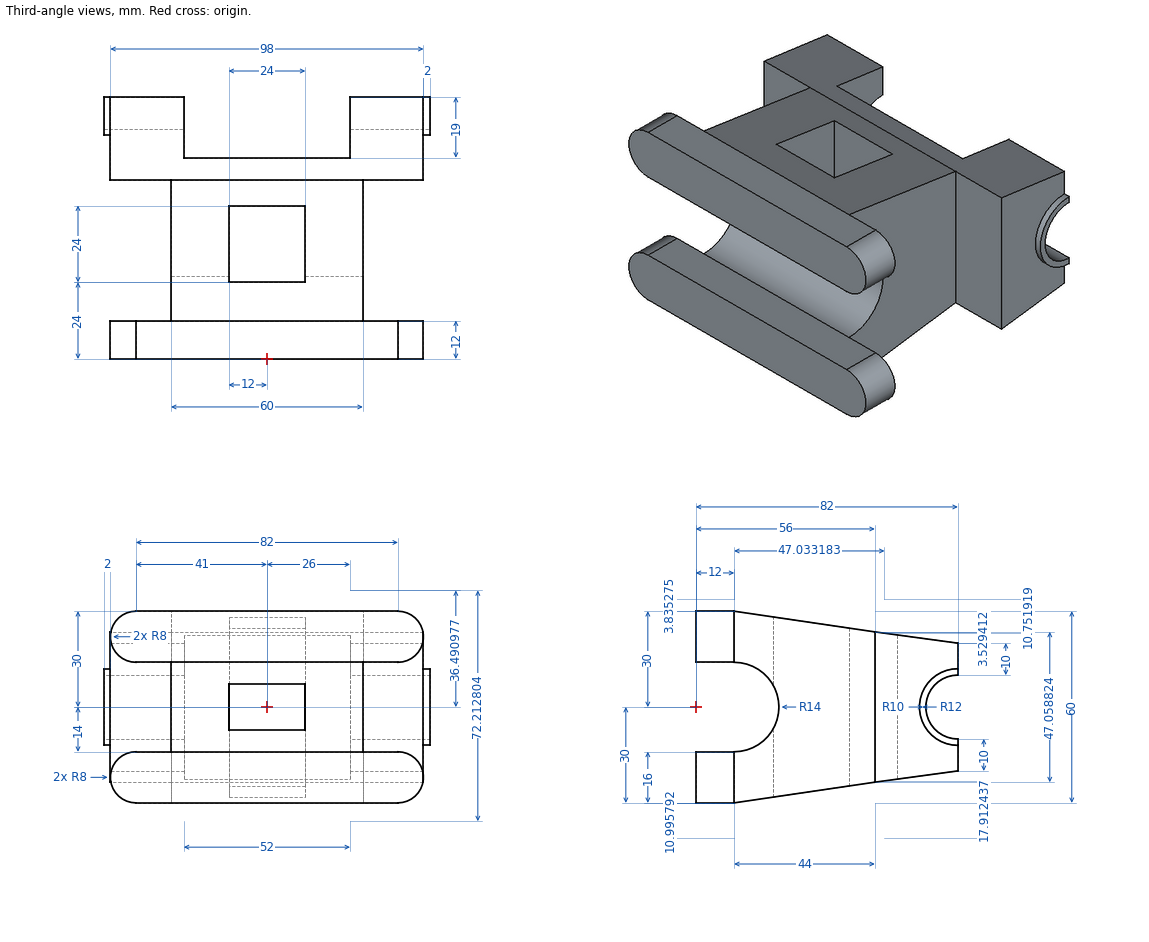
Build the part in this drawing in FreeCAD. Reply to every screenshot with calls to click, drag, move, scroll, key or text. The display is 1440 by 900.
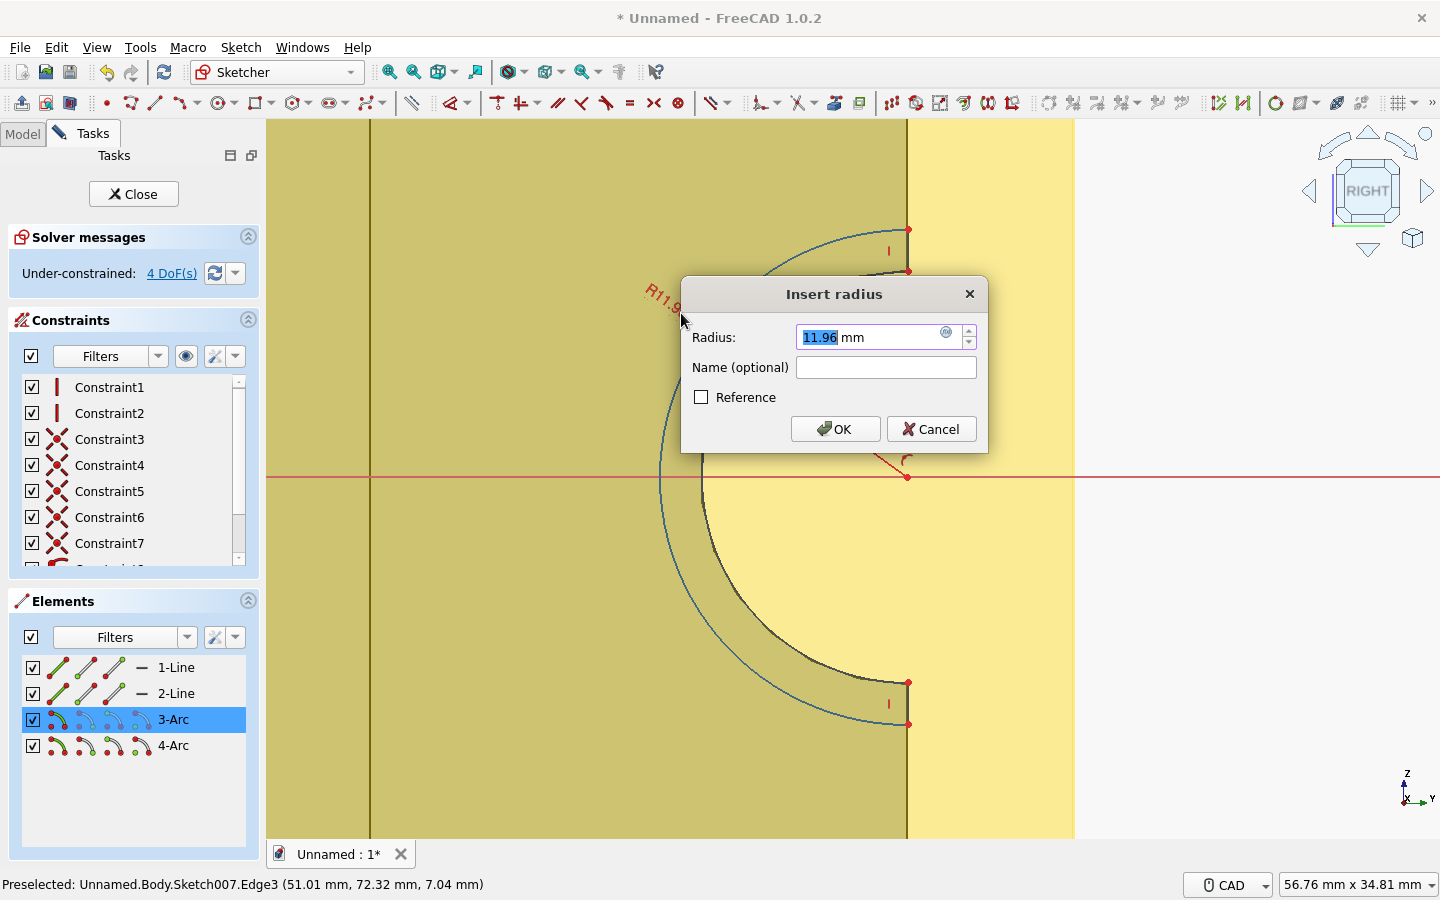
text(12)
key(Return)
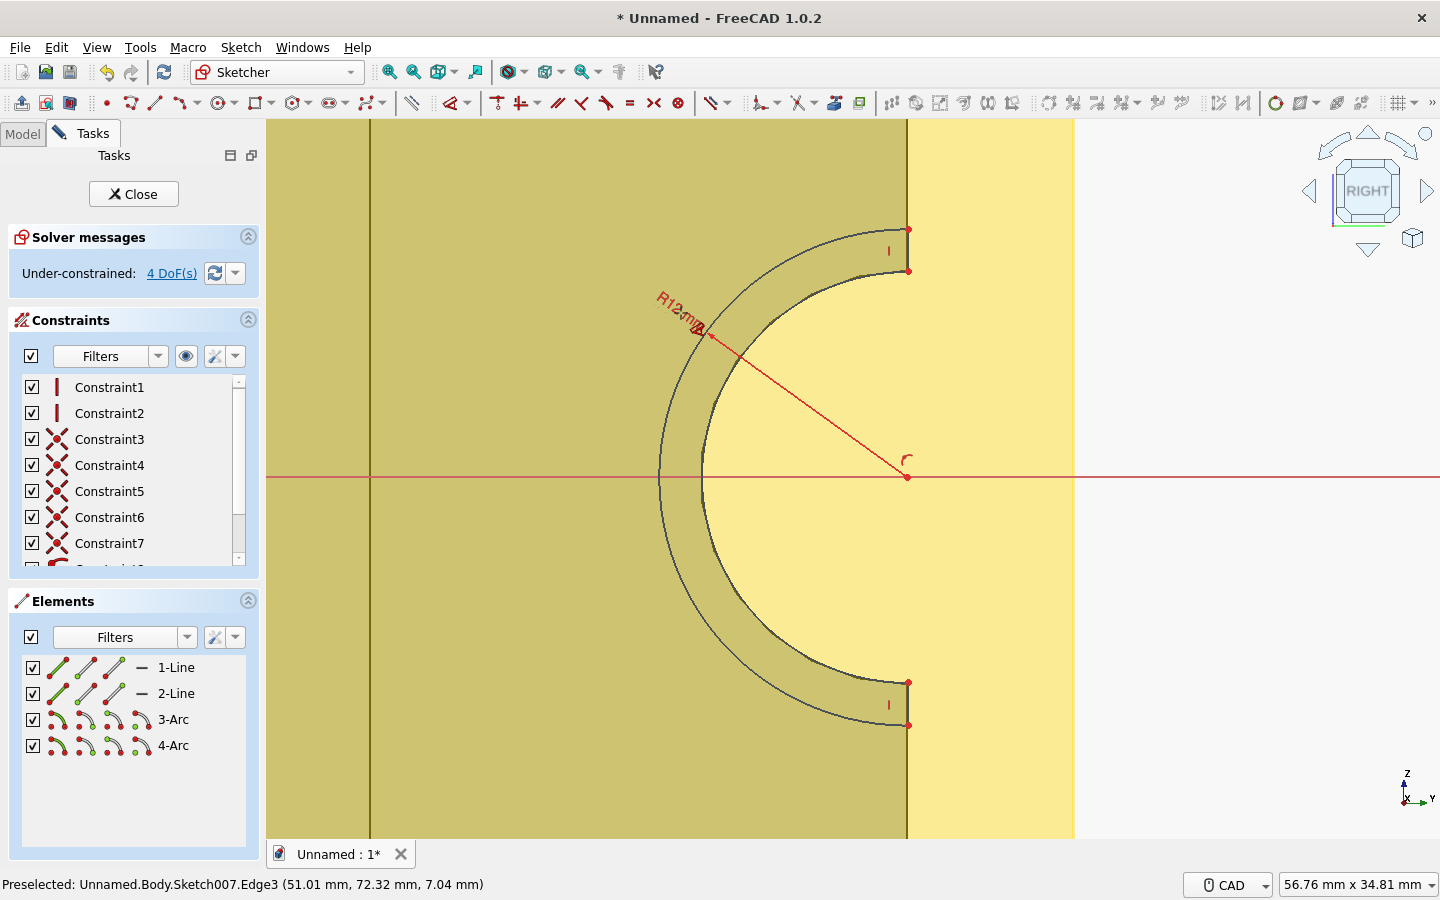
click(741, 357)
click(1047, 285)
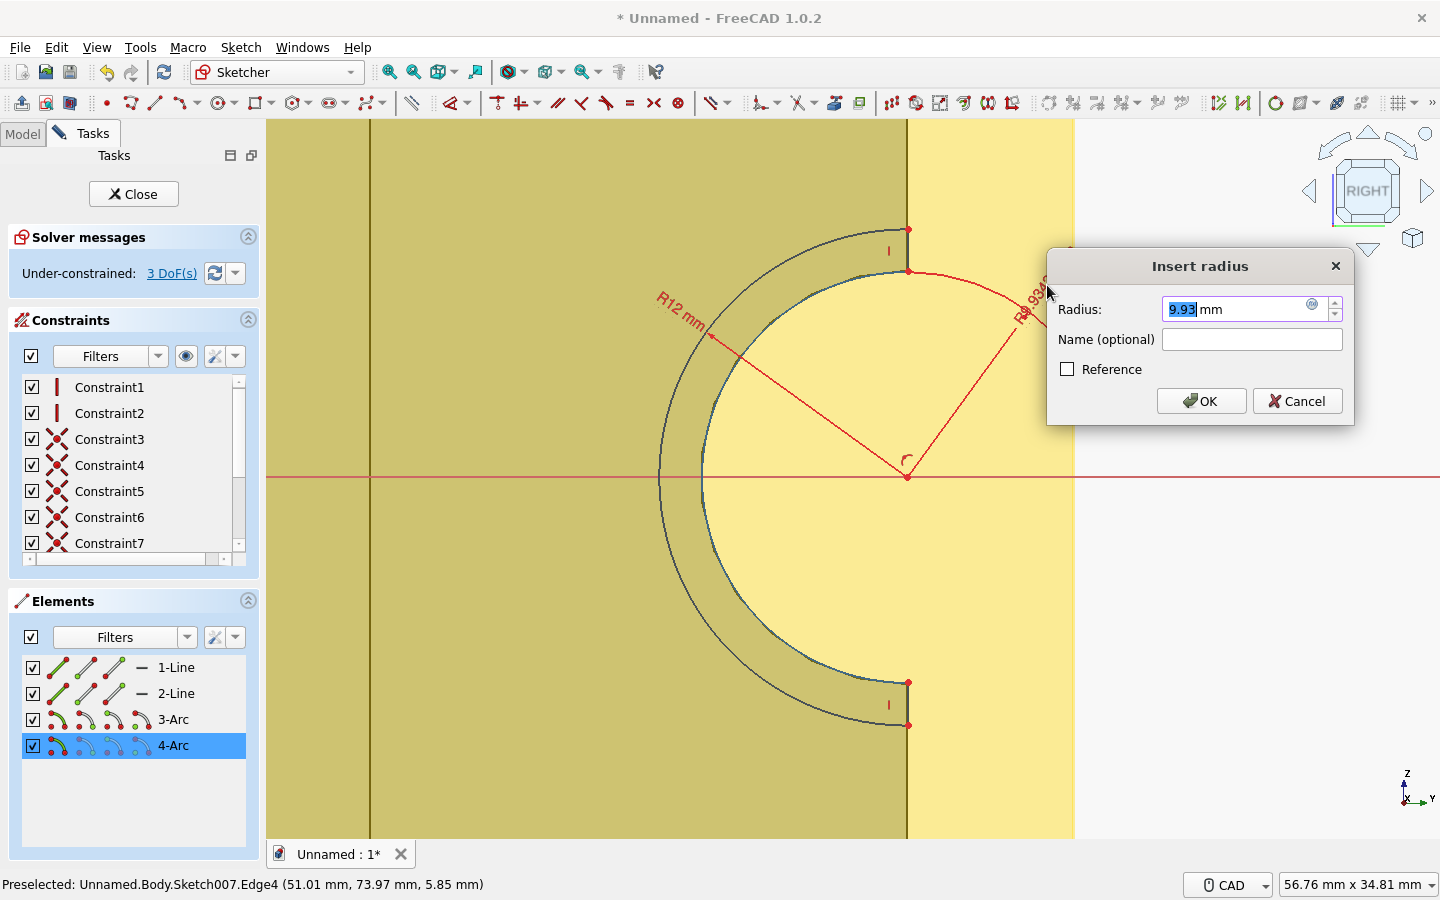
text(10)
key(Return)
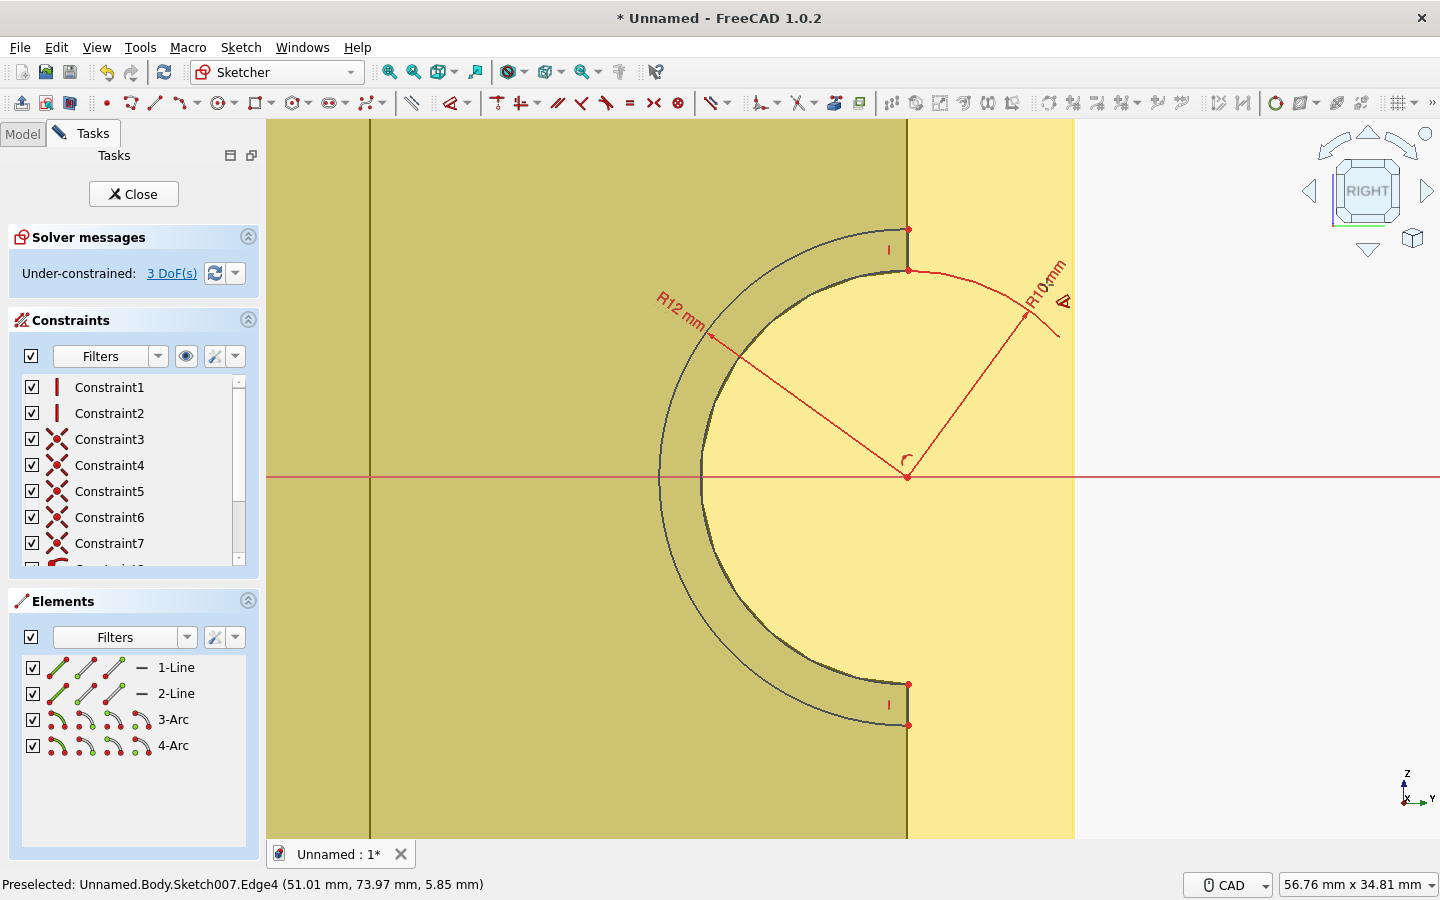
click(908, 271)
click(601, 237)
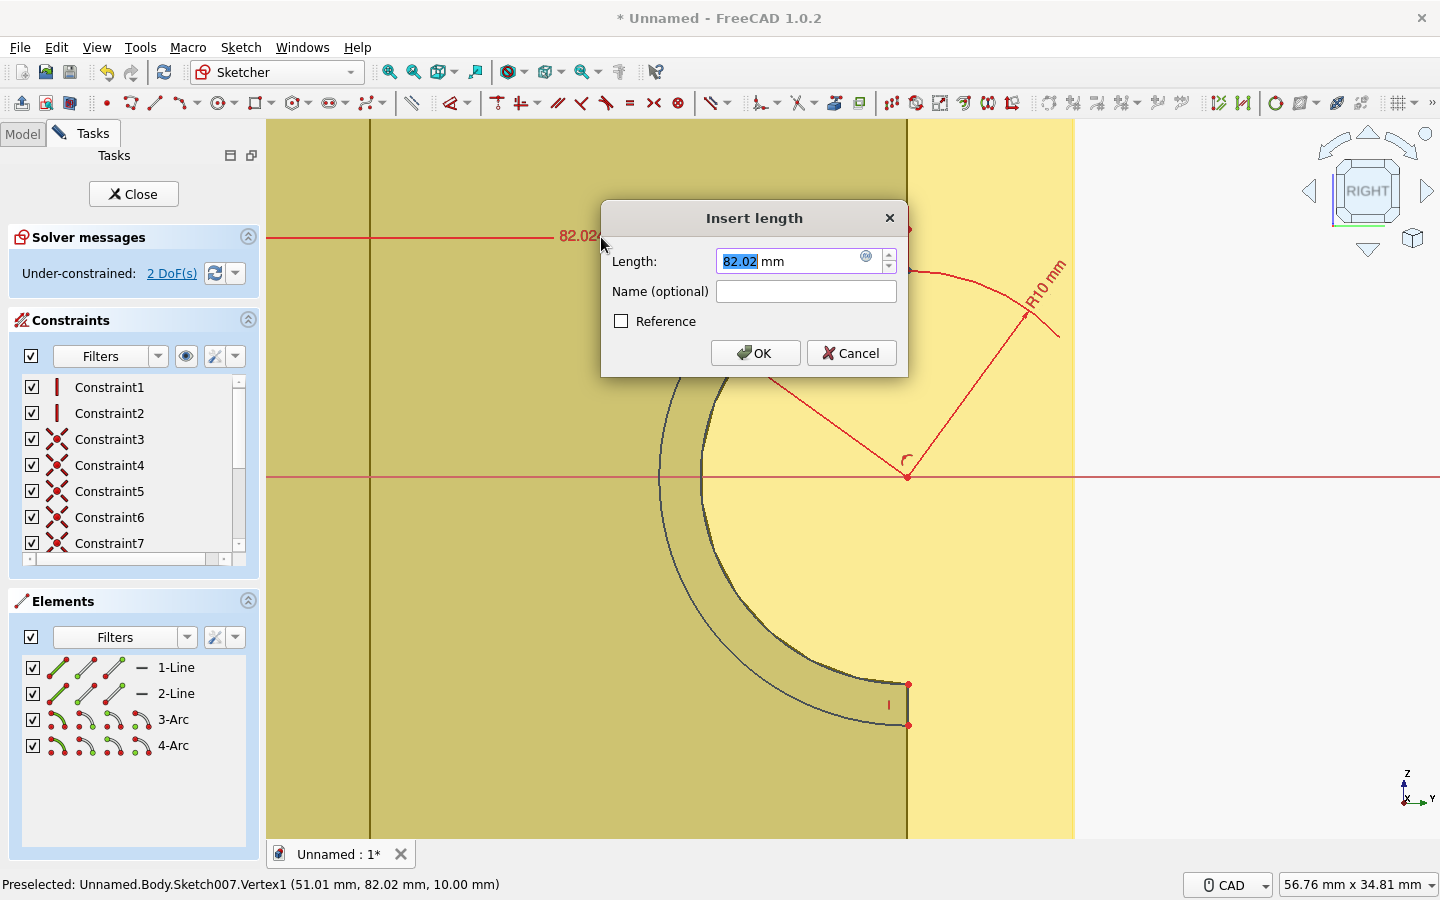
text(82)
key(Return)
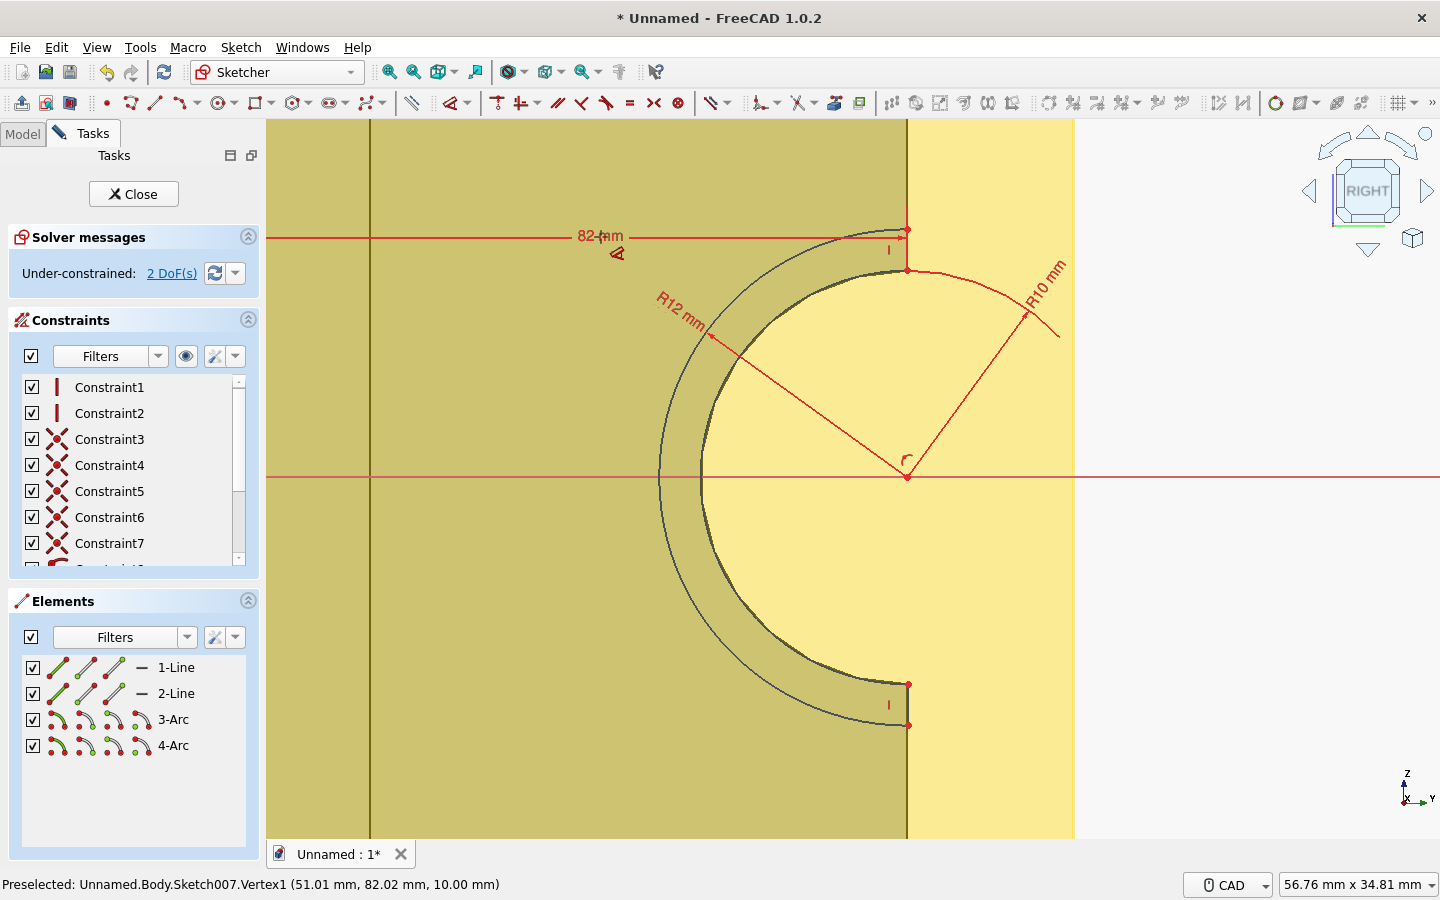
click(908, 726)
click(601, 760)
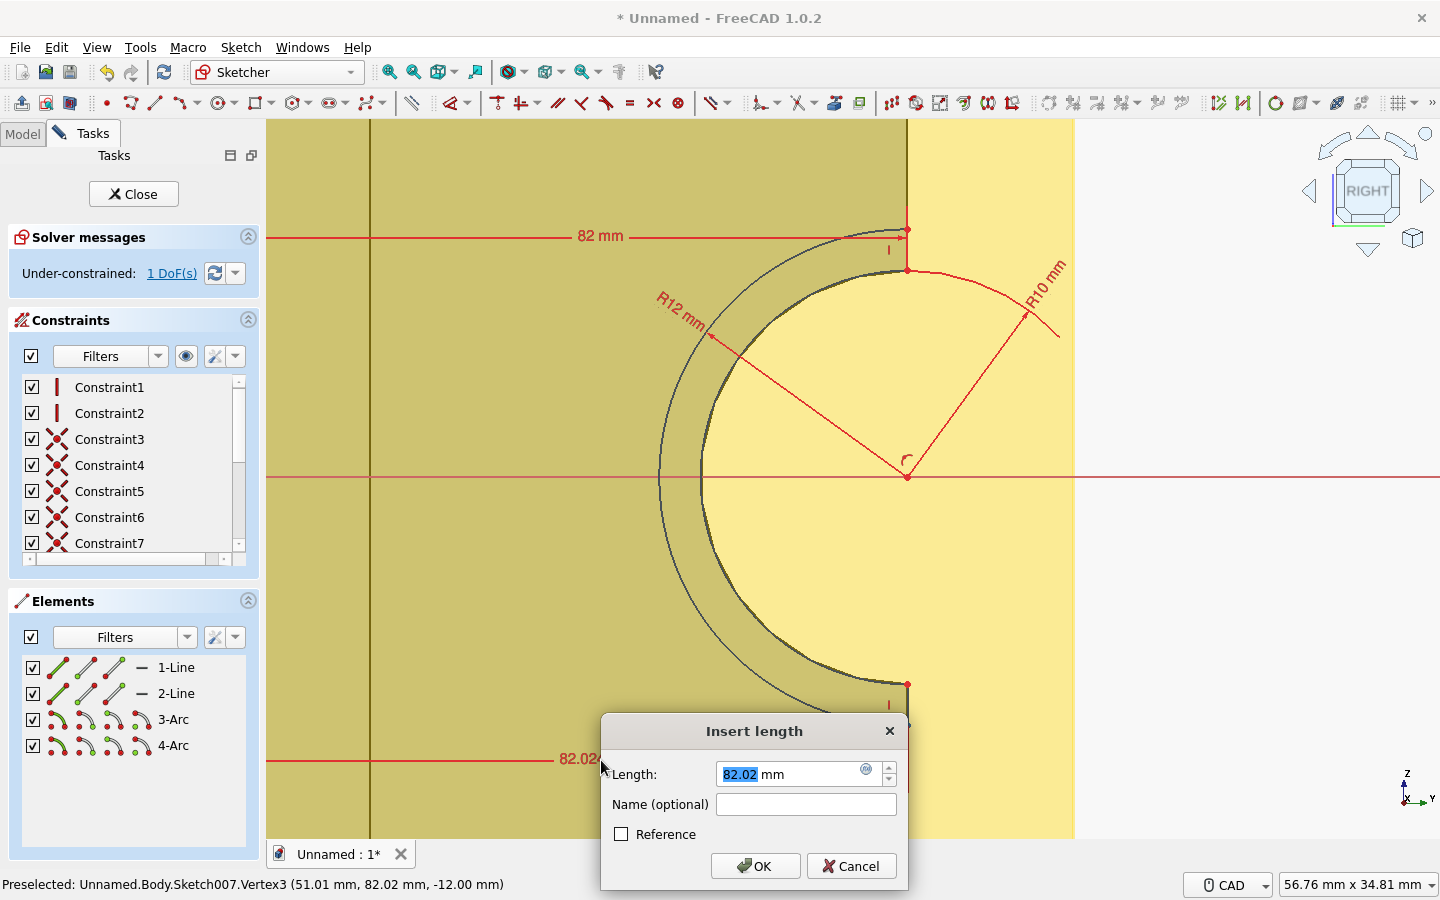
text(82)
key(Return)